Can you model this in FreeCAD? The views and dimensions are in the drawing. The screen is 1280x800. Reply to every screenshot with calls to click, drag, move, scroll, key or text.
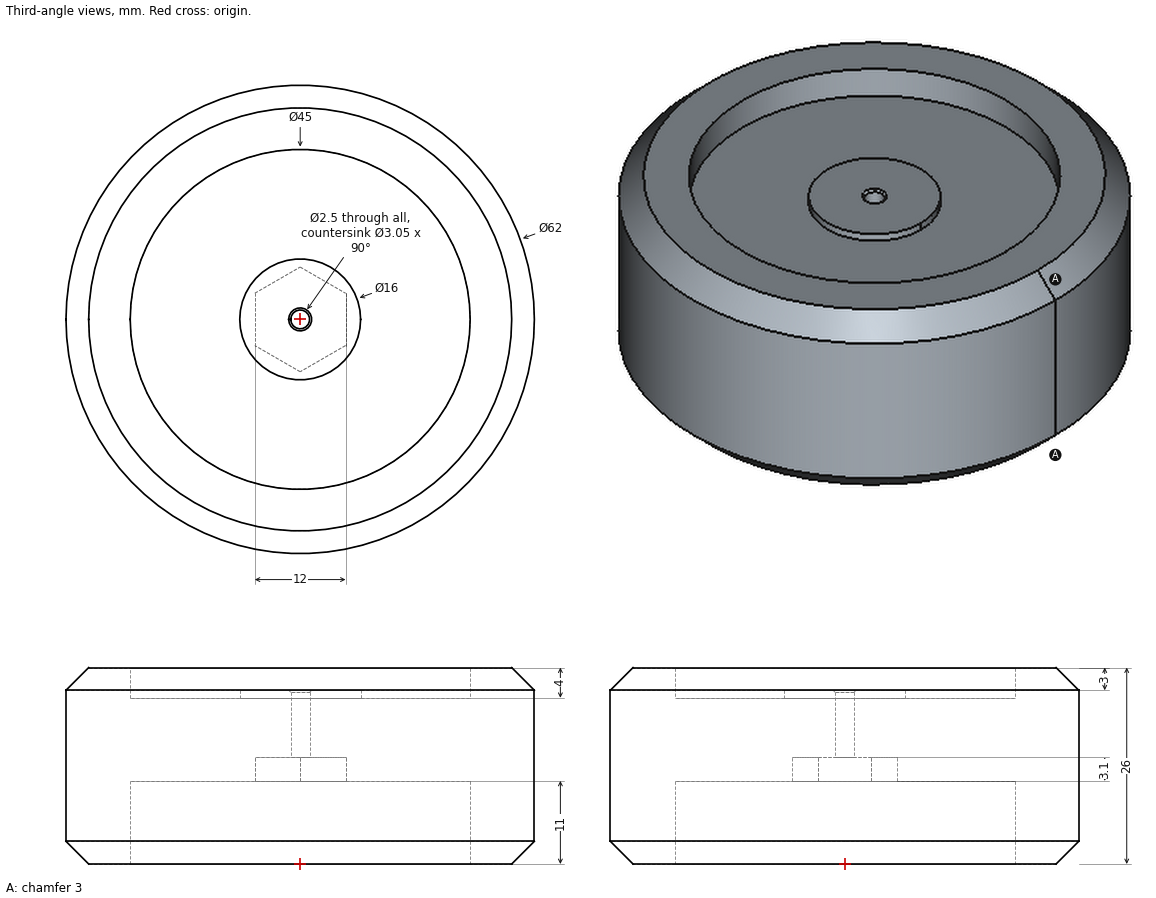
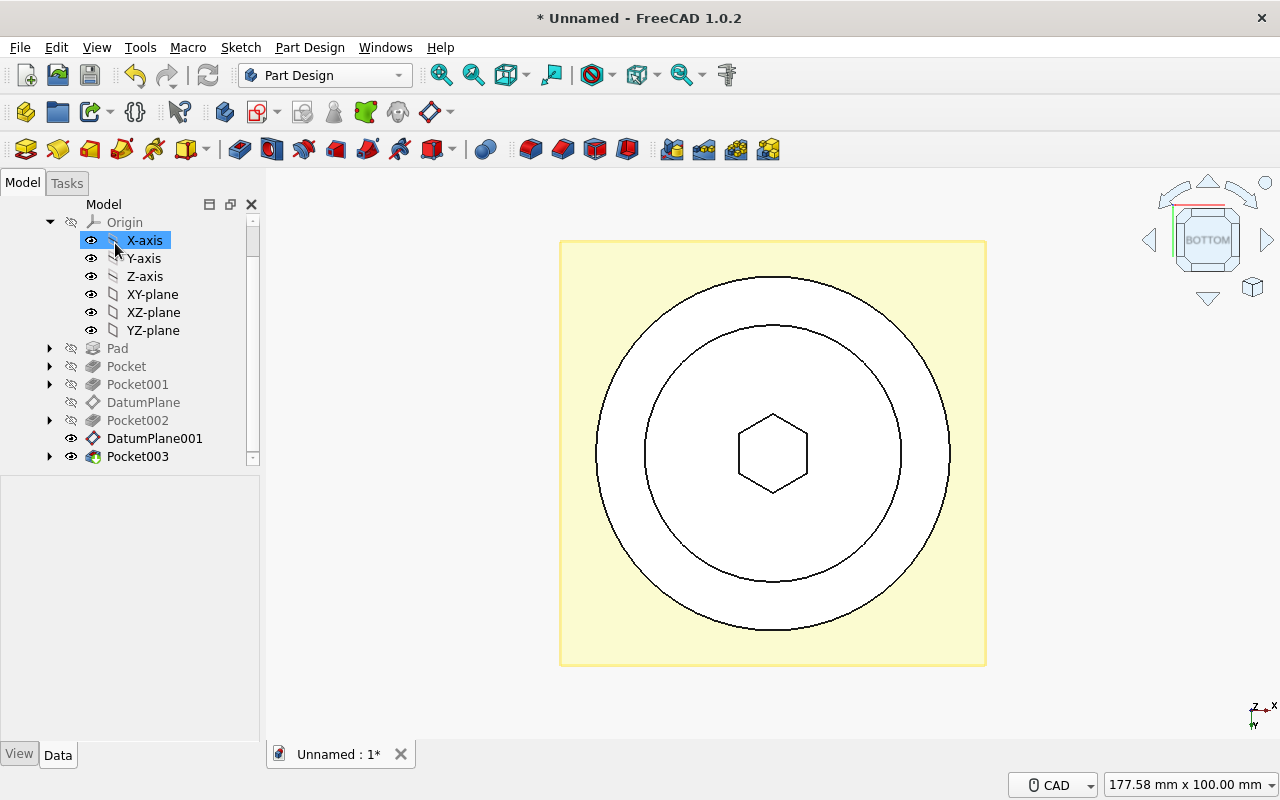
click(116, 438)
key(space)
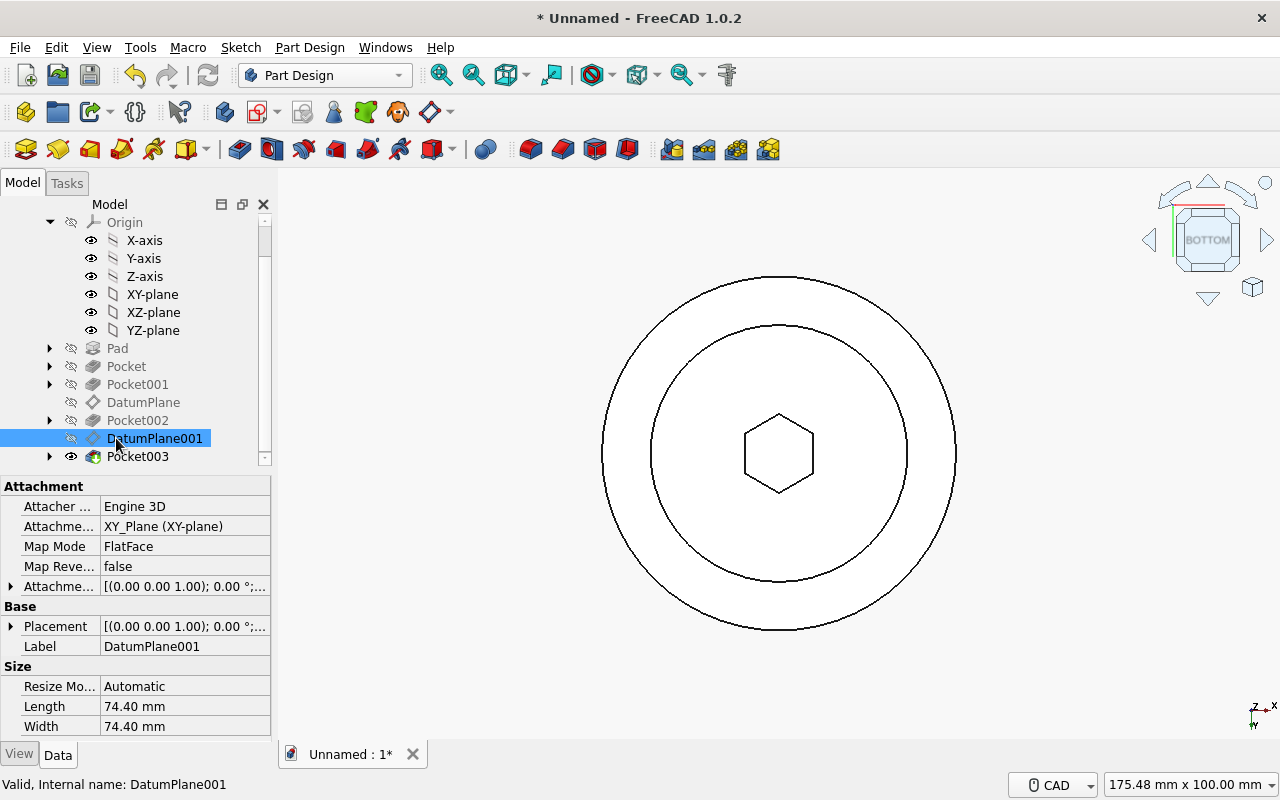
key(0)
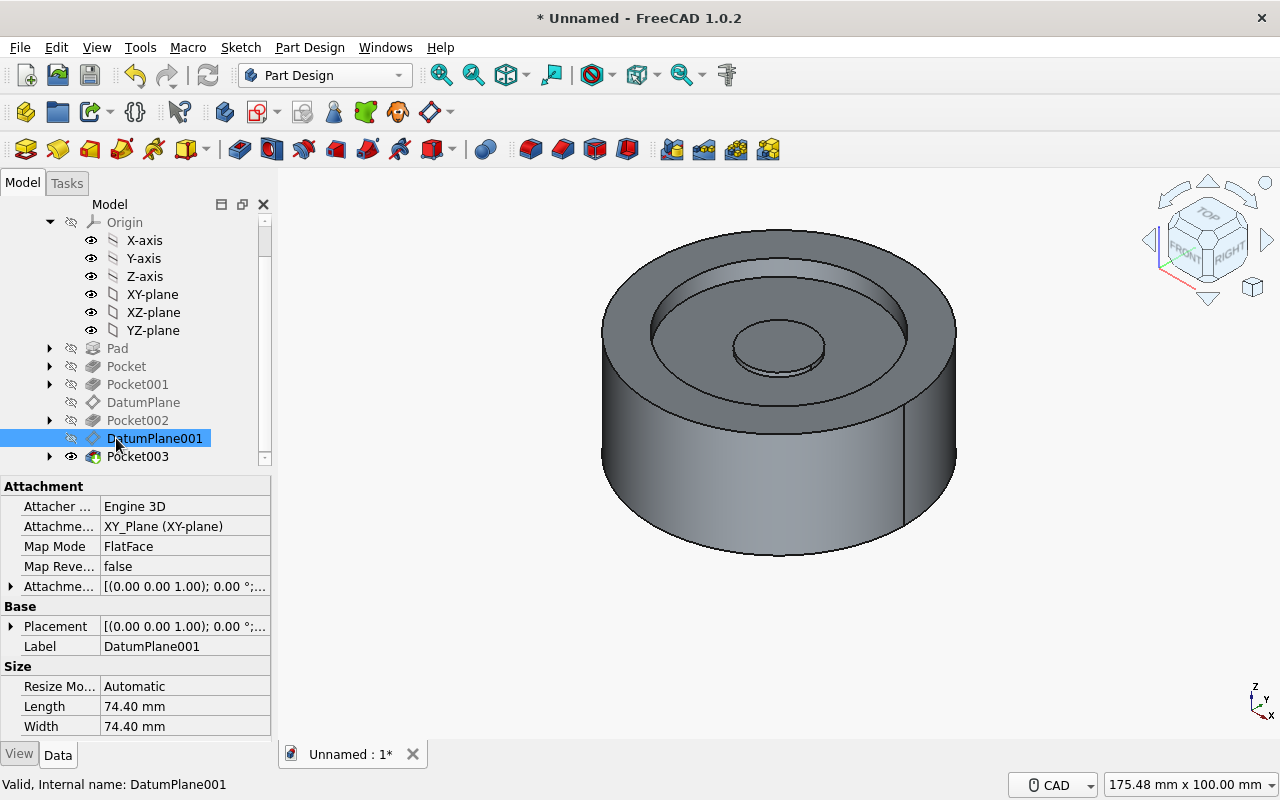
click(779, 345)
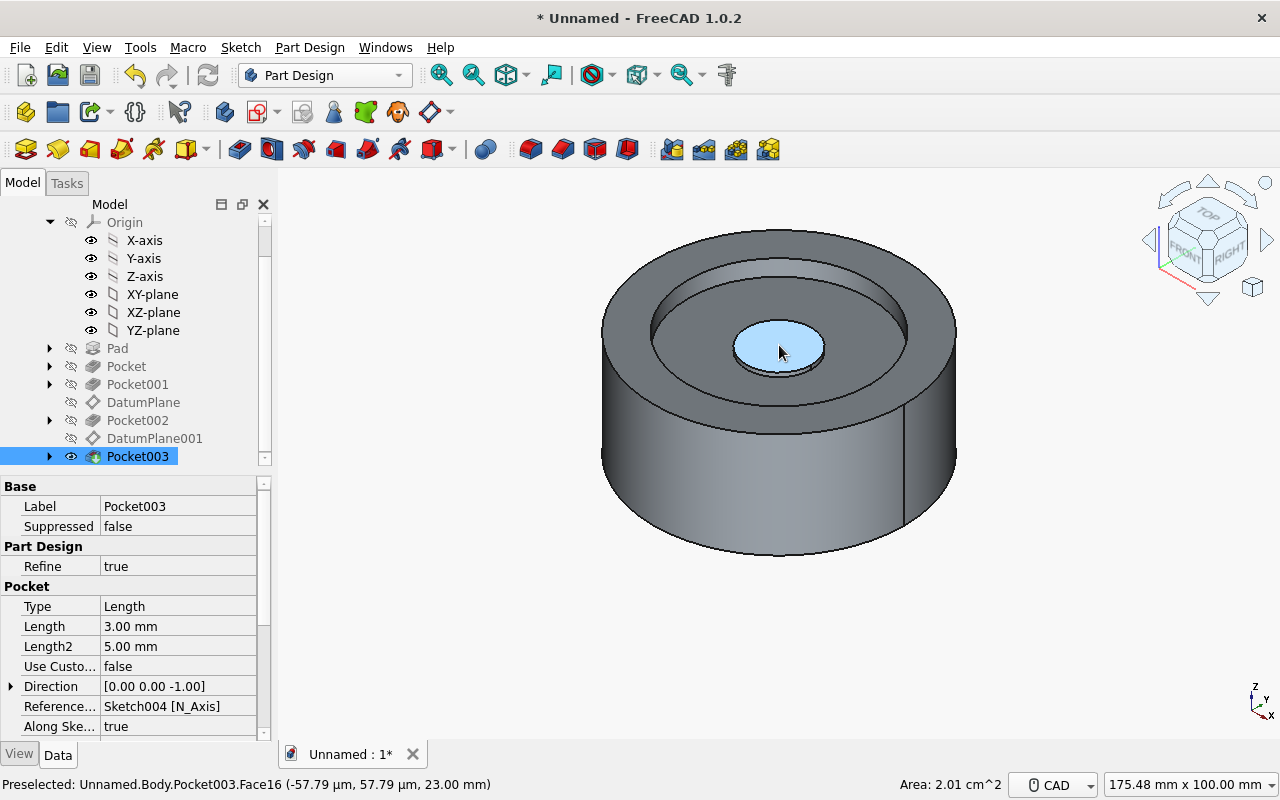
click(258, 112)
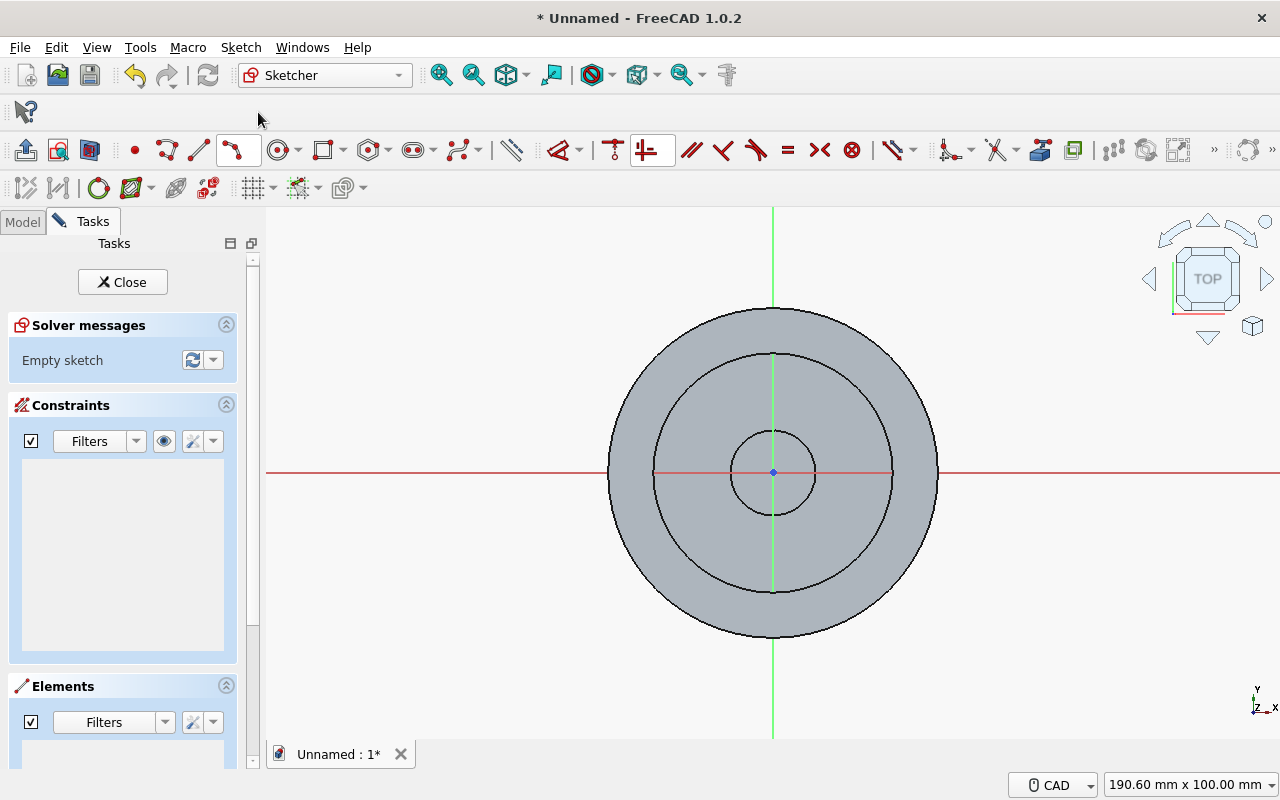
scroll(777, 473, up, 15)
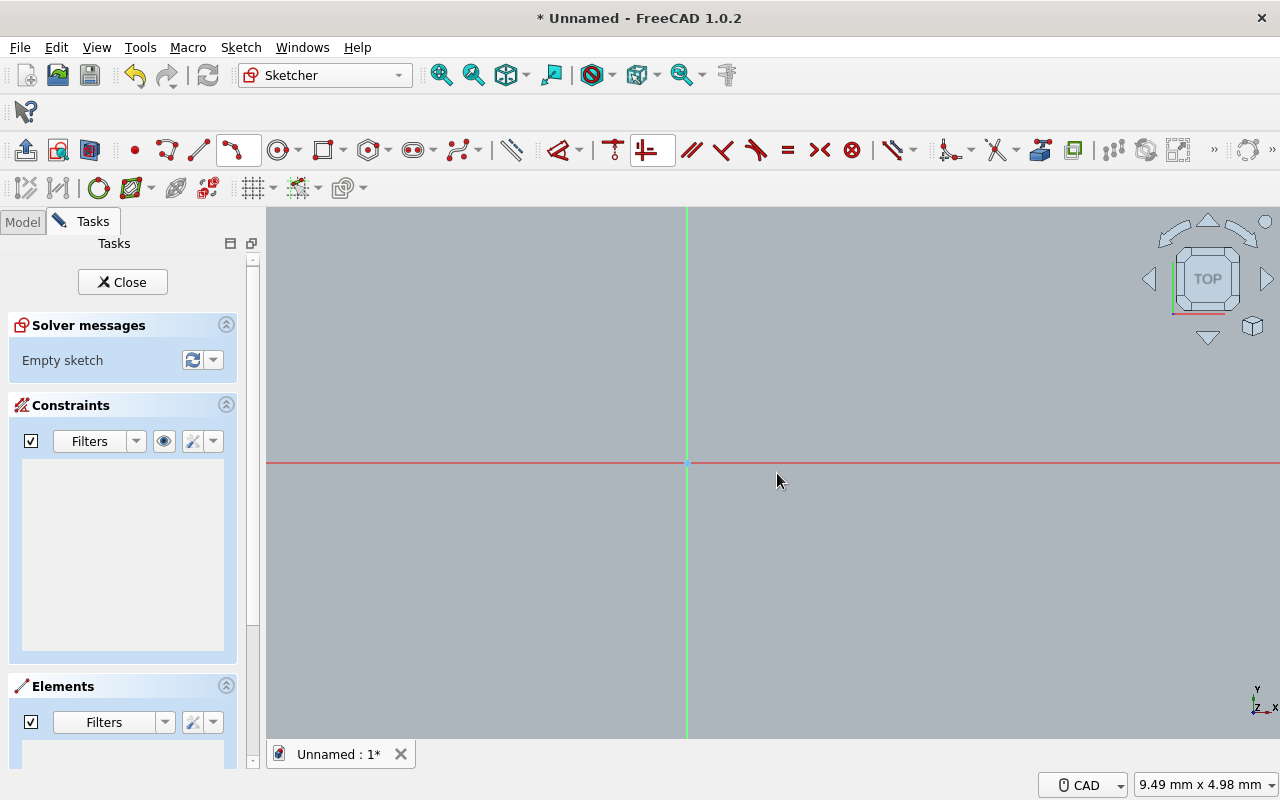
click(278, 150)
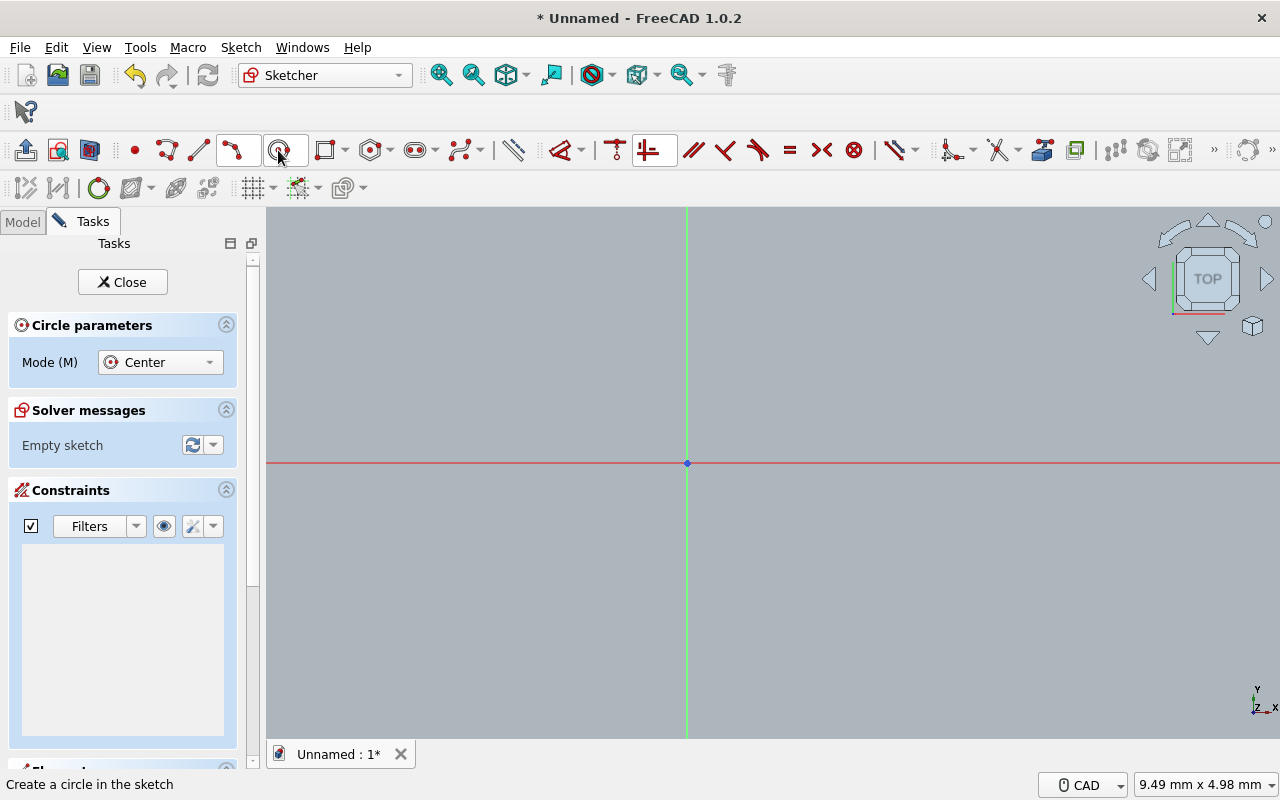
click(687, 463)
click(781, 369)
key(Escape)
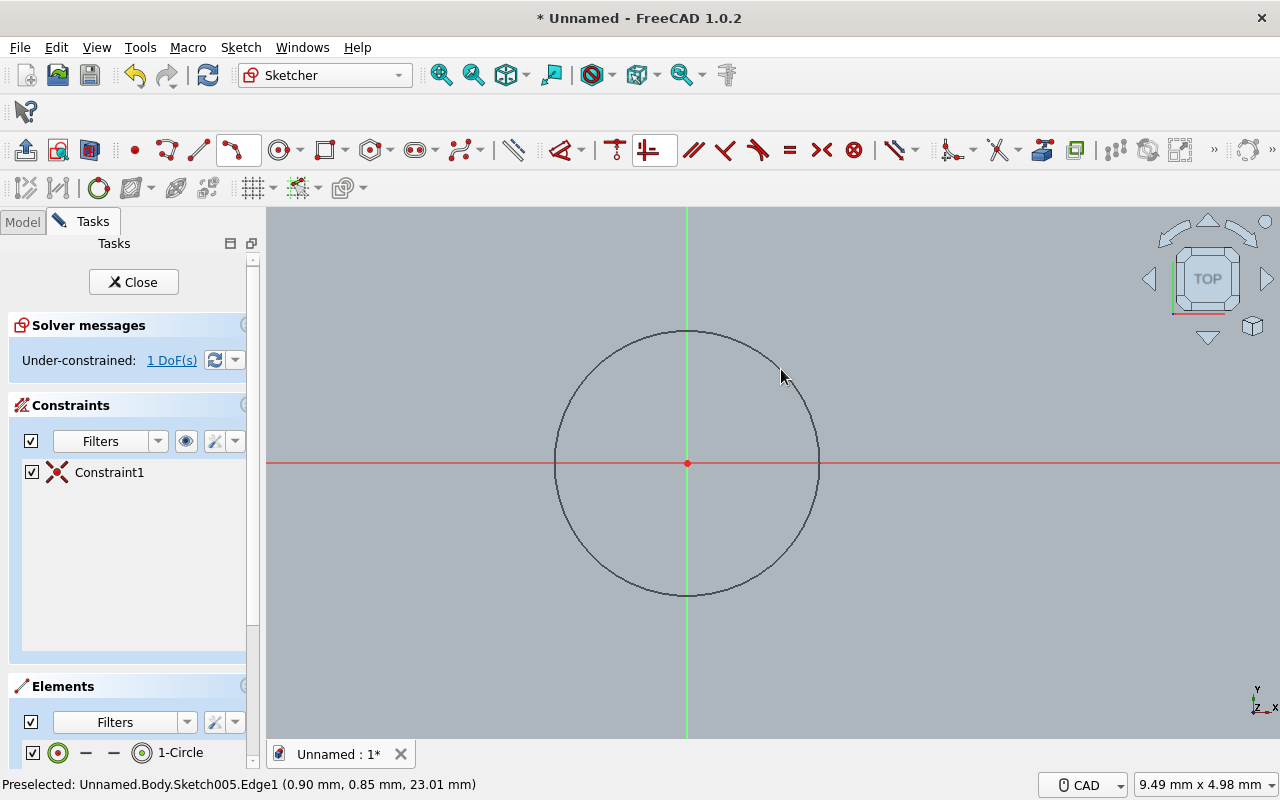
click(560, 150)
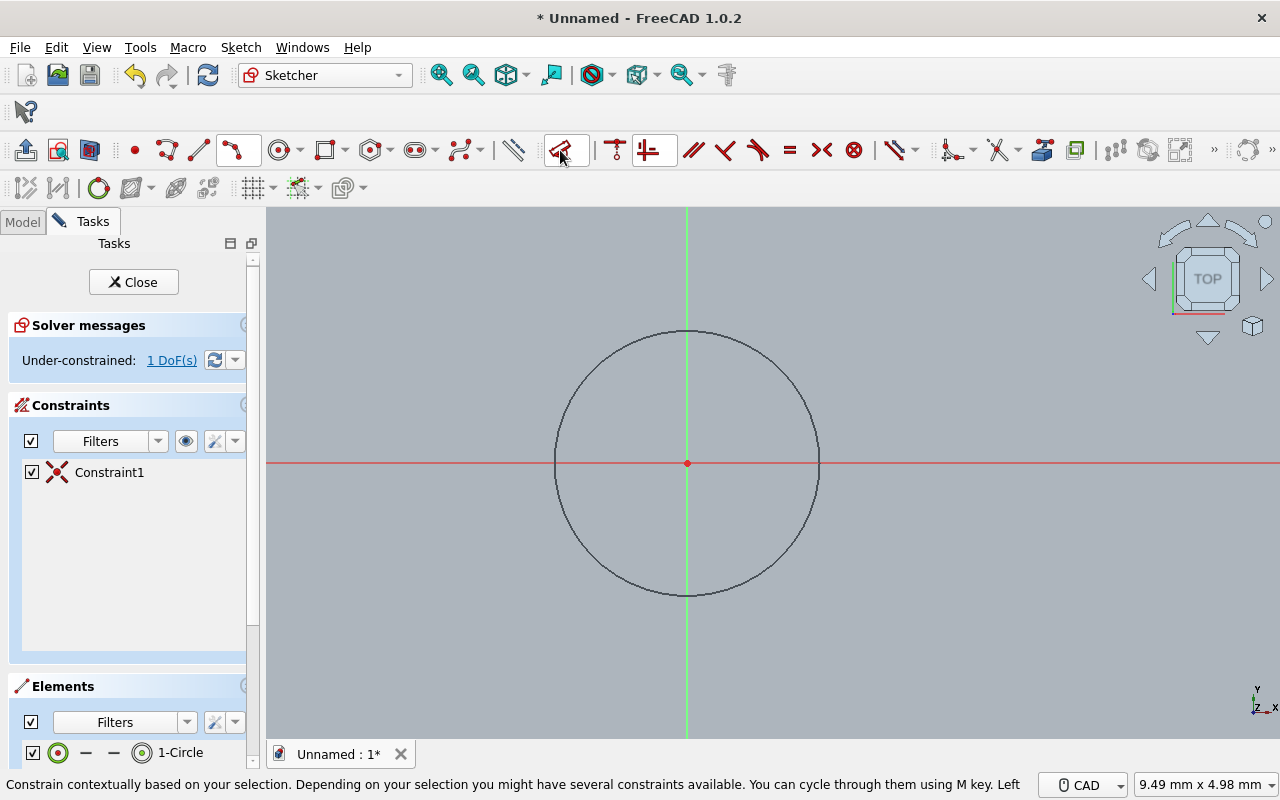
click(780, 369)
click(802, 346)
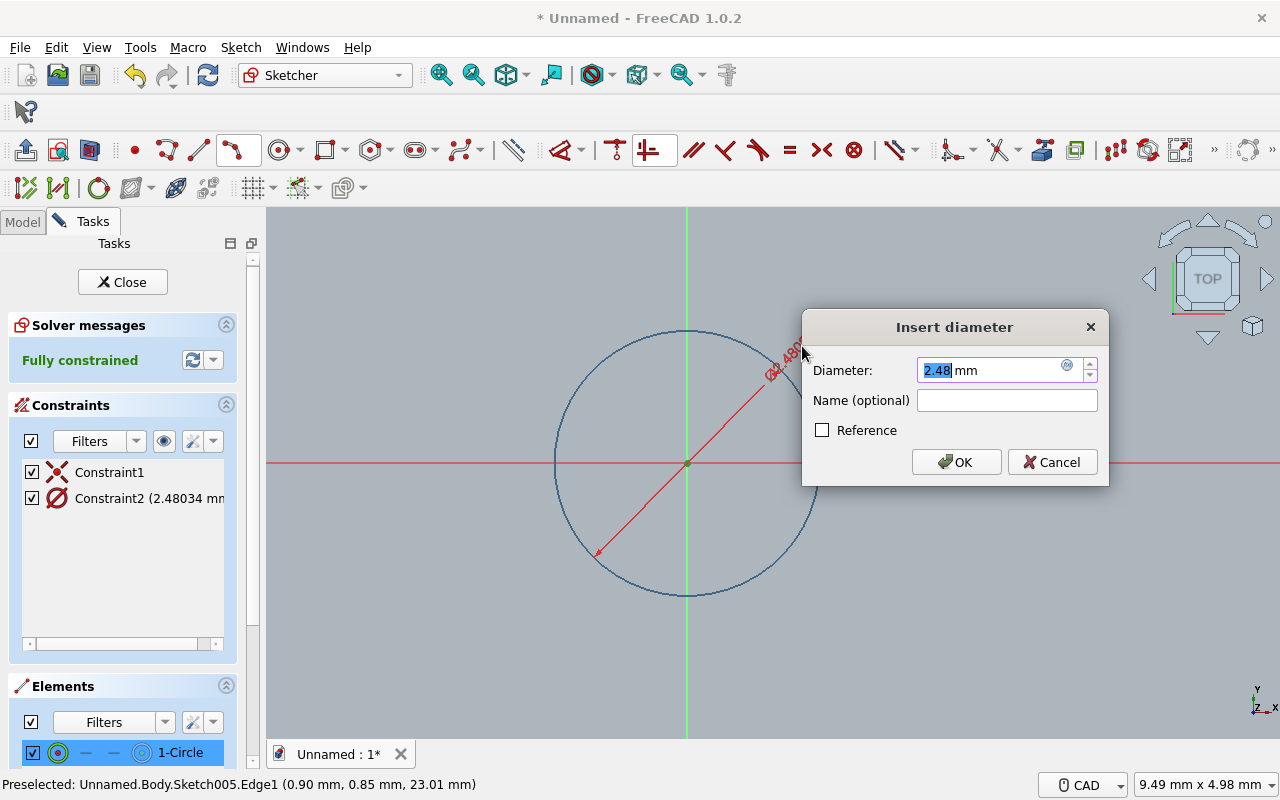
text(2.5)
key(Return)
key(Escape)